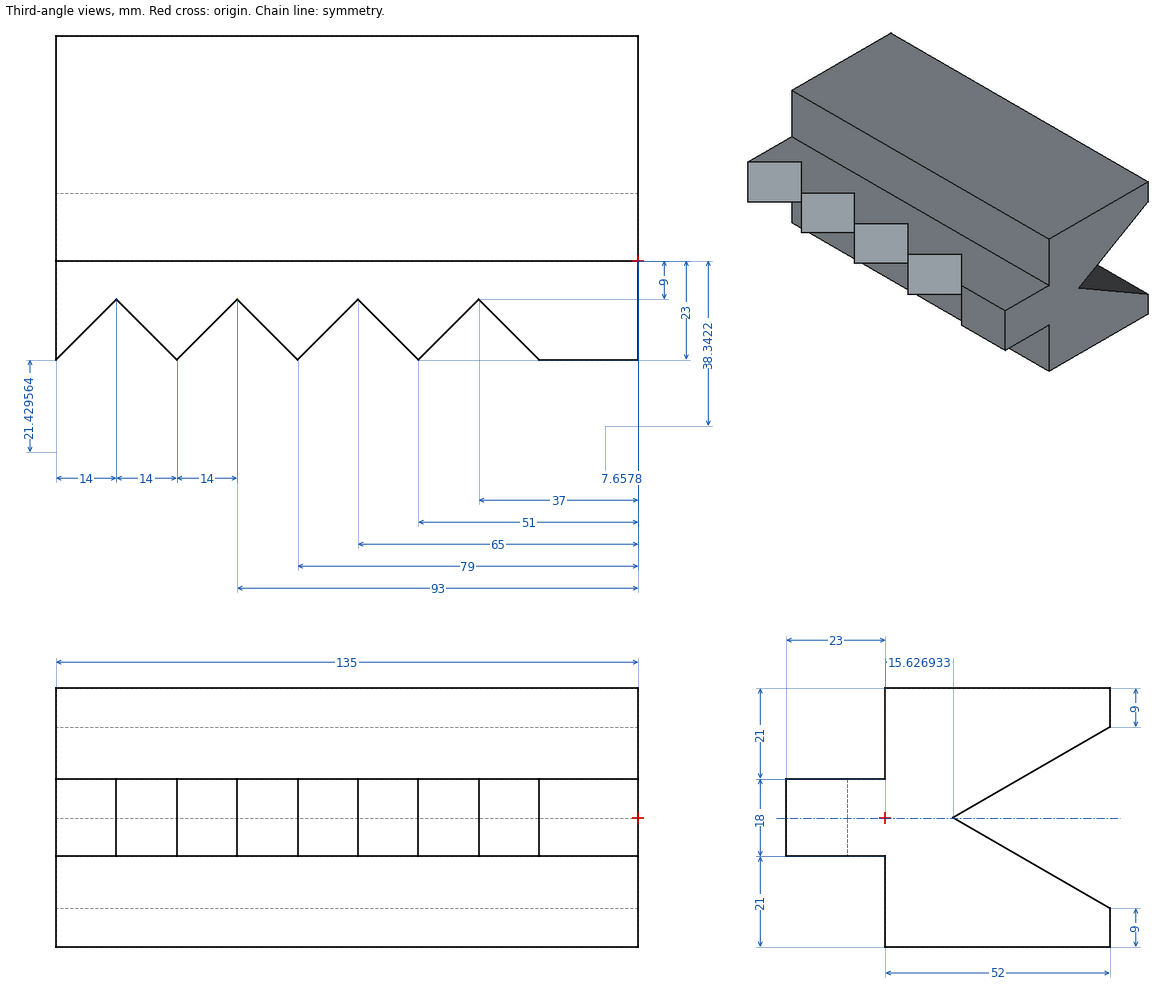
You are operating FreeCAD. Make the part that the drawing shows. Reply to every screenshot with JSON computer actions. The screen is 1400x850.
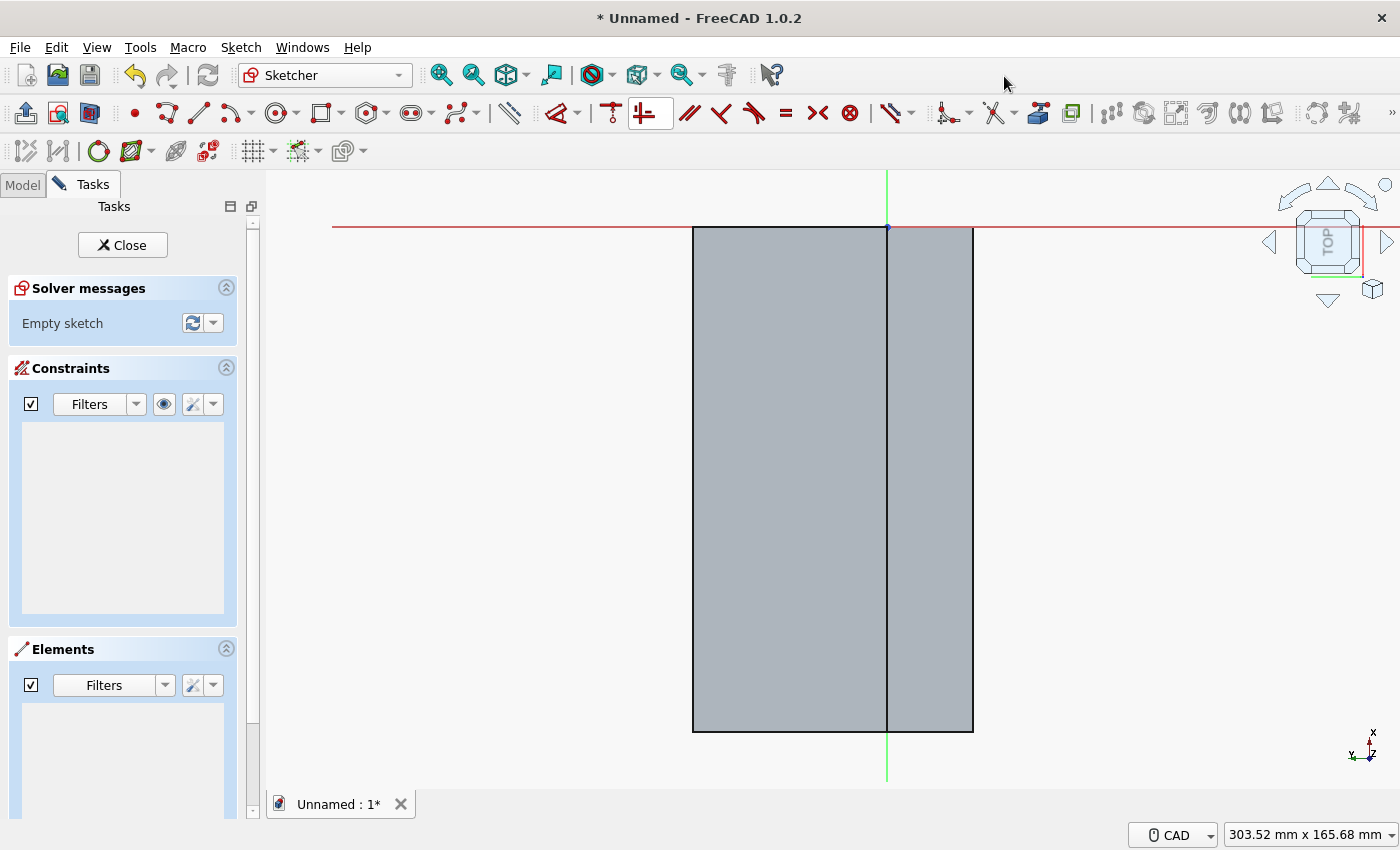
{"action": "left_click", "coordinate": [90, 114]}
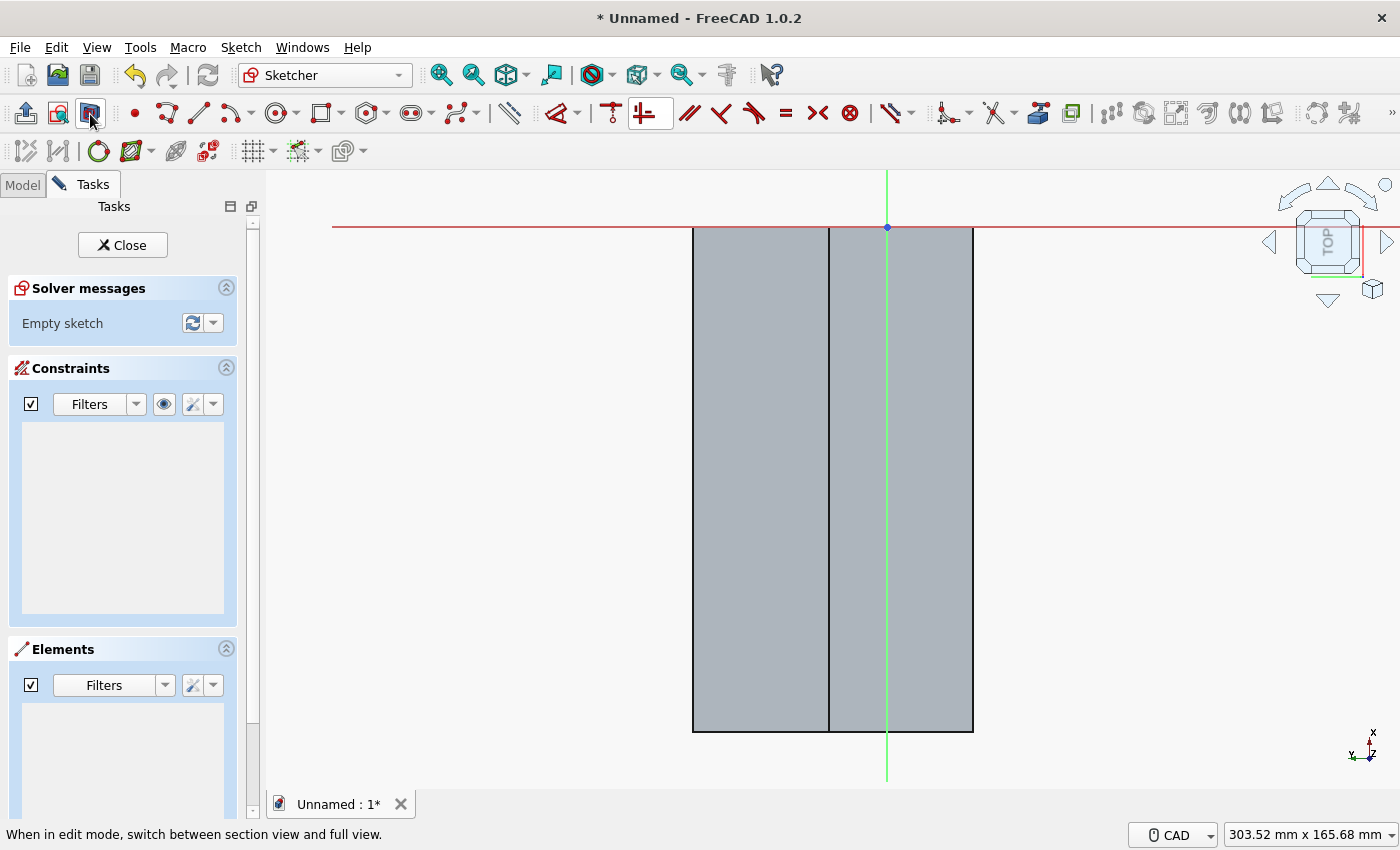
{"action": "left_click", "coordinate": [168, 114]}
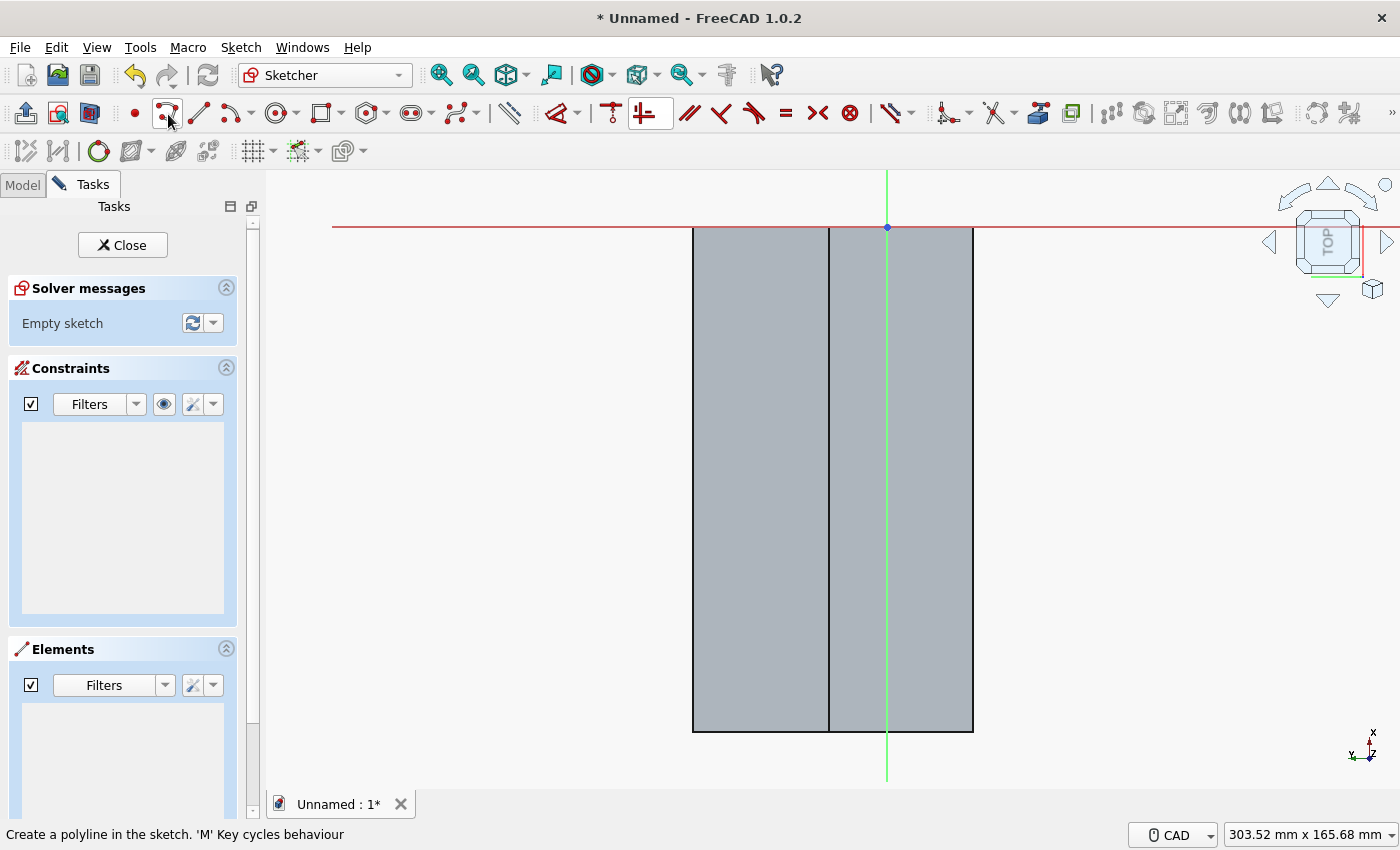
{"action": "left_click", "coordinate": [921, 366]}
{"action": "left_click", "coordinate": [973, 418]}
{"action": "left_click", "coordinate": [921, 470]}
{"action": "left_click", "coordinate": [973, 522]}
{"action": "left_click", "coordinate": [921, 575]}
{"action": "left_click", "coordinate": [973, 627]}
{"action": "left_click", "coordinate": [921, 679]}
{"action": "left_click", "coordinate": [973, 732]}
{"action": "left_click", "coordinate": [1053, 732]}
{"action": "left_click", "coordinate": [1030, 256]}
{"action": "left_click", "coordinate": [921, 367]}
{"action": "key", "text": "Escape"}
{"action": "key", "text": "Escape"}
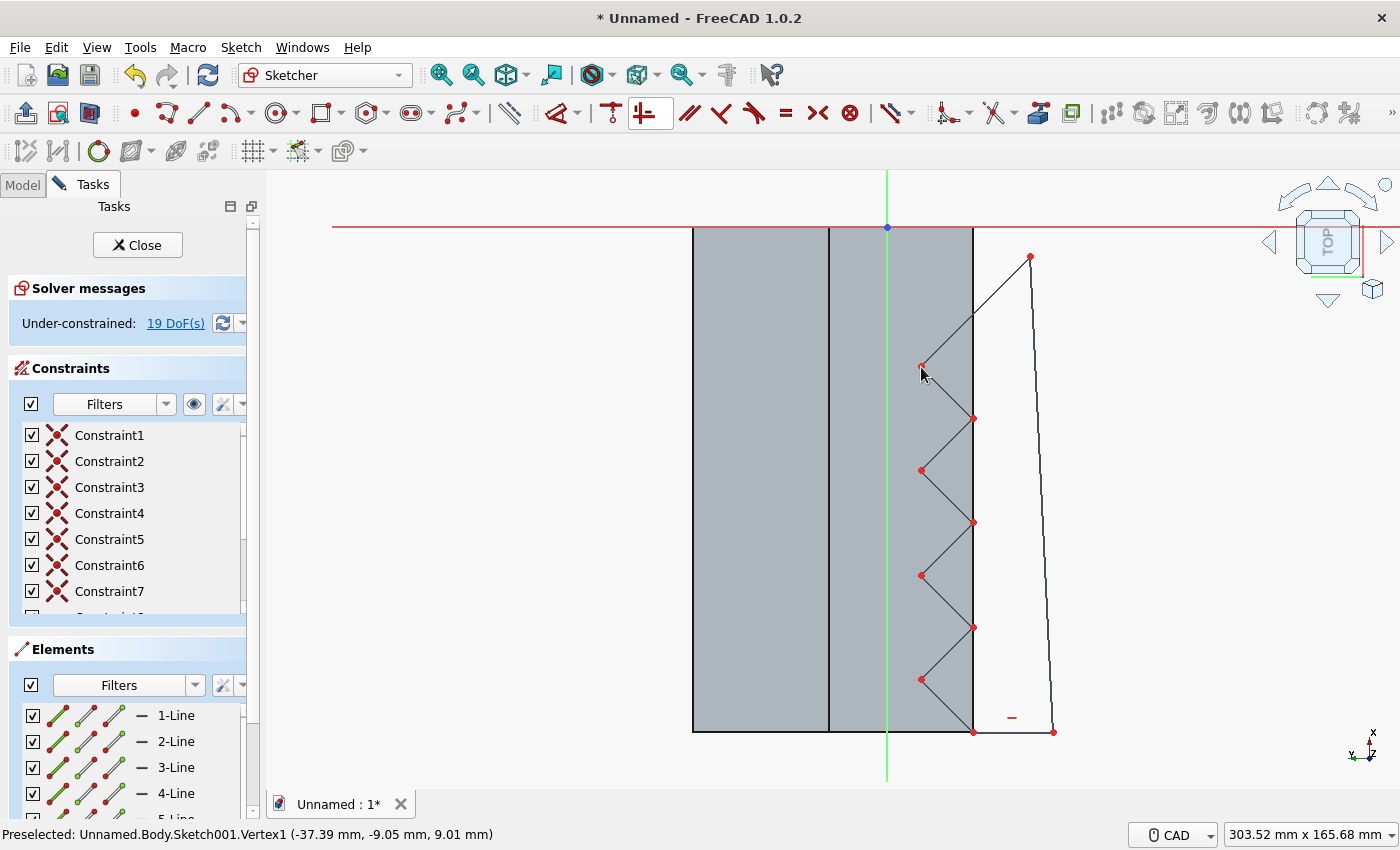
{"action": "left_click", "coordinate": [556, 114]}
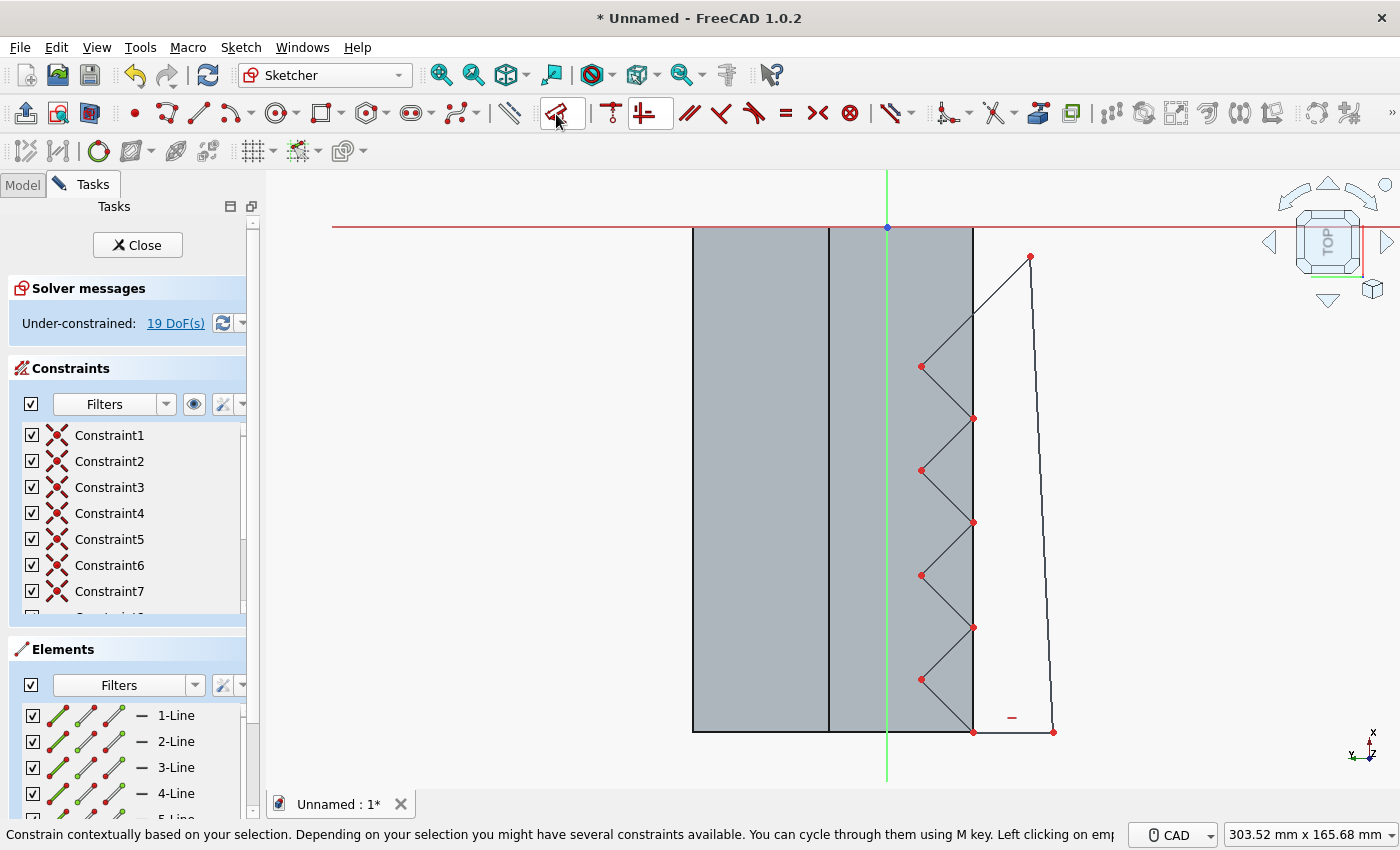
{"action": "left_click", "coordinate": [921, 367]}
{"action": "left_click", "coordinate": [904, 401]}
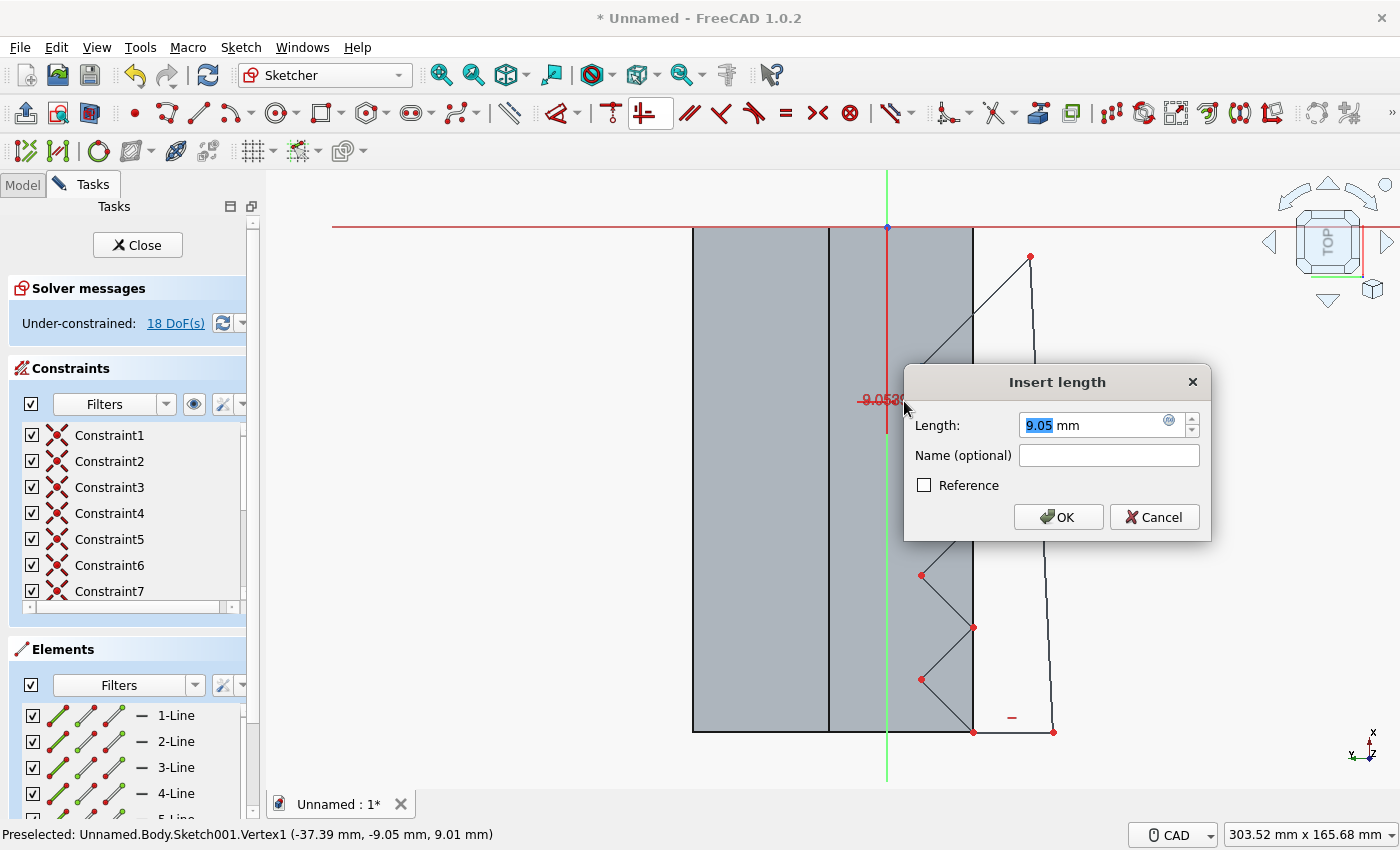
{"action": "type", "text": "9"}
{"action": "key", "text": "Return"}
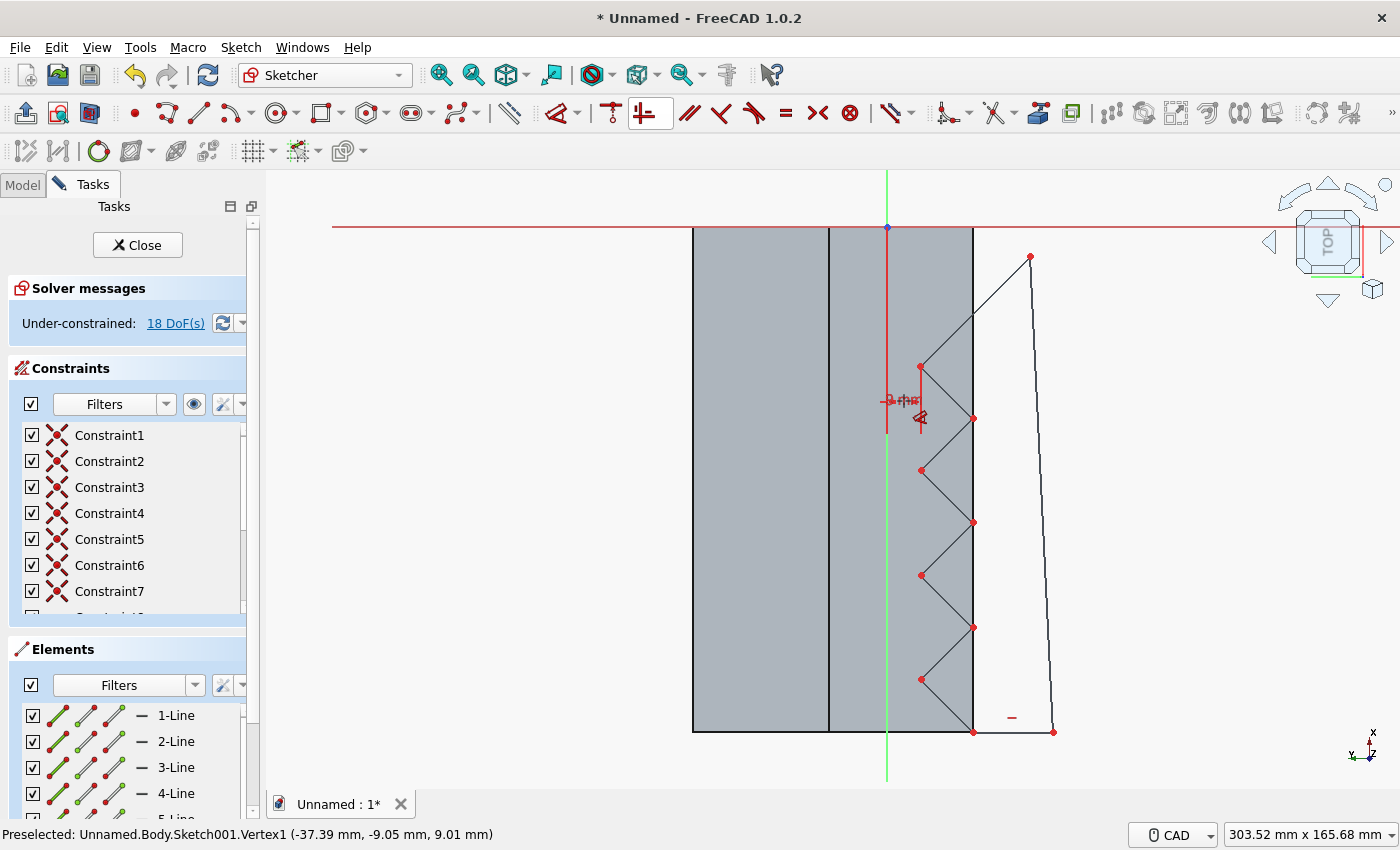
{"action": "left_click", "coordinate": [921, 471]}
{"action": "left_click", "coordinate": [904, 505]}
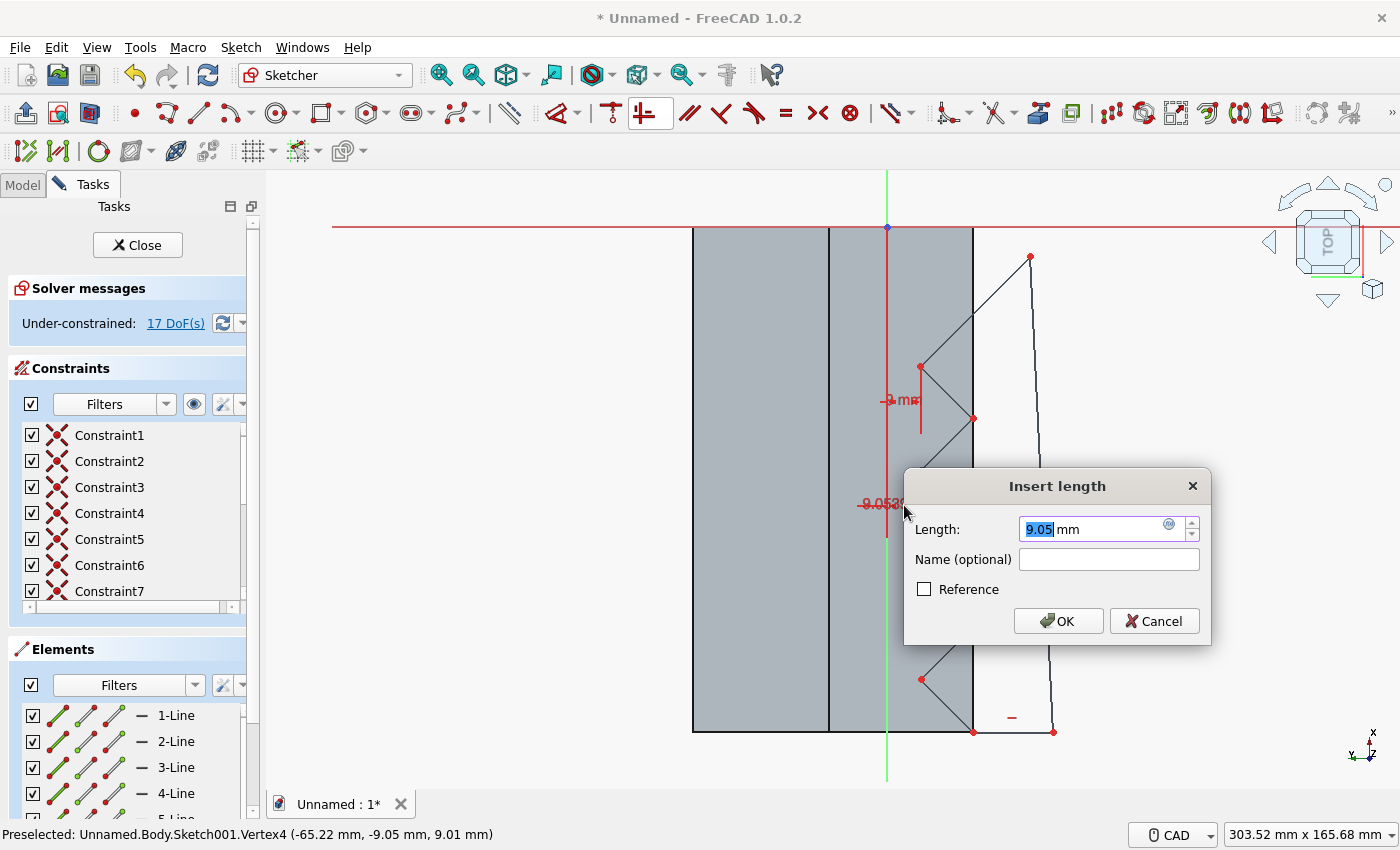
{"action": "type", "text": "9"}
{"action": "key", "text": "Return"}